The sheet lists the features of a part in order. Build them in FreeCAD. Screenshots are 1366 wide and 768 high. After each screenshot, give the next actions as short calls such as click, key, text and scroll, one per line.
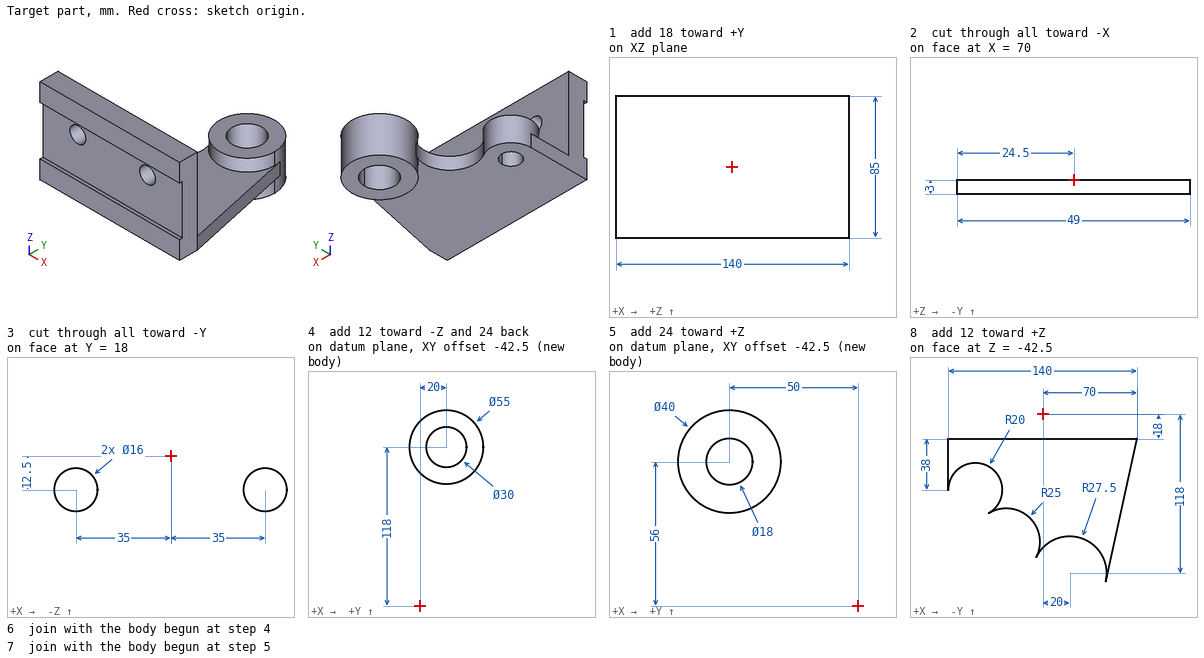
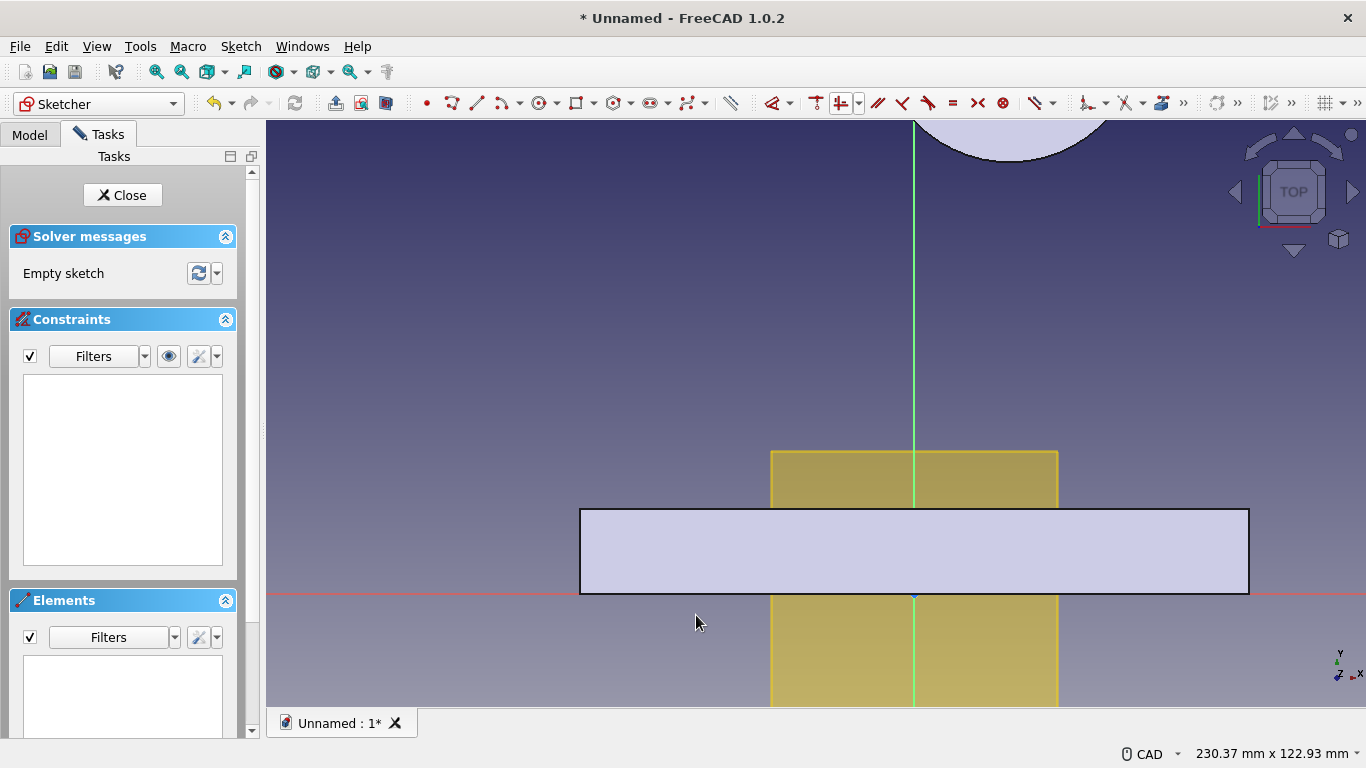
click(538, 104)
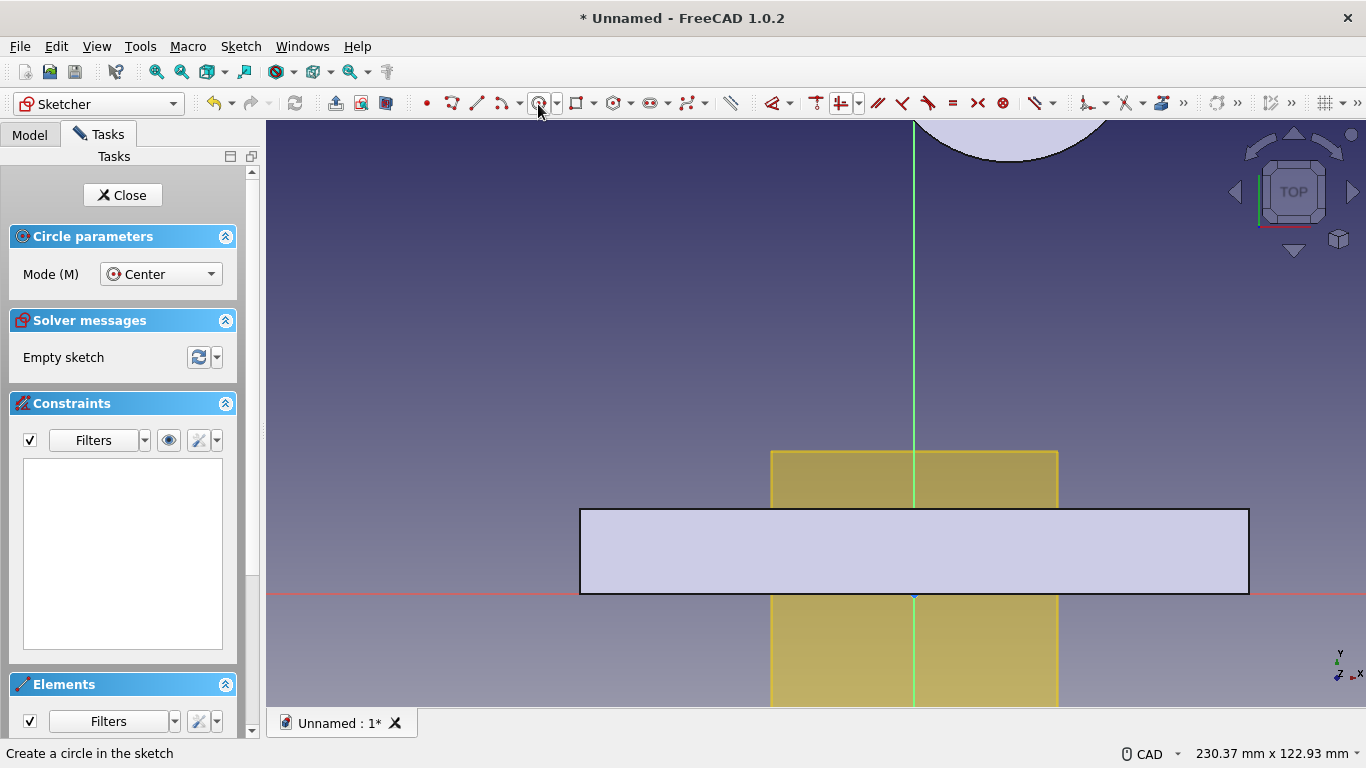
click(676, 327)
click(743, 260)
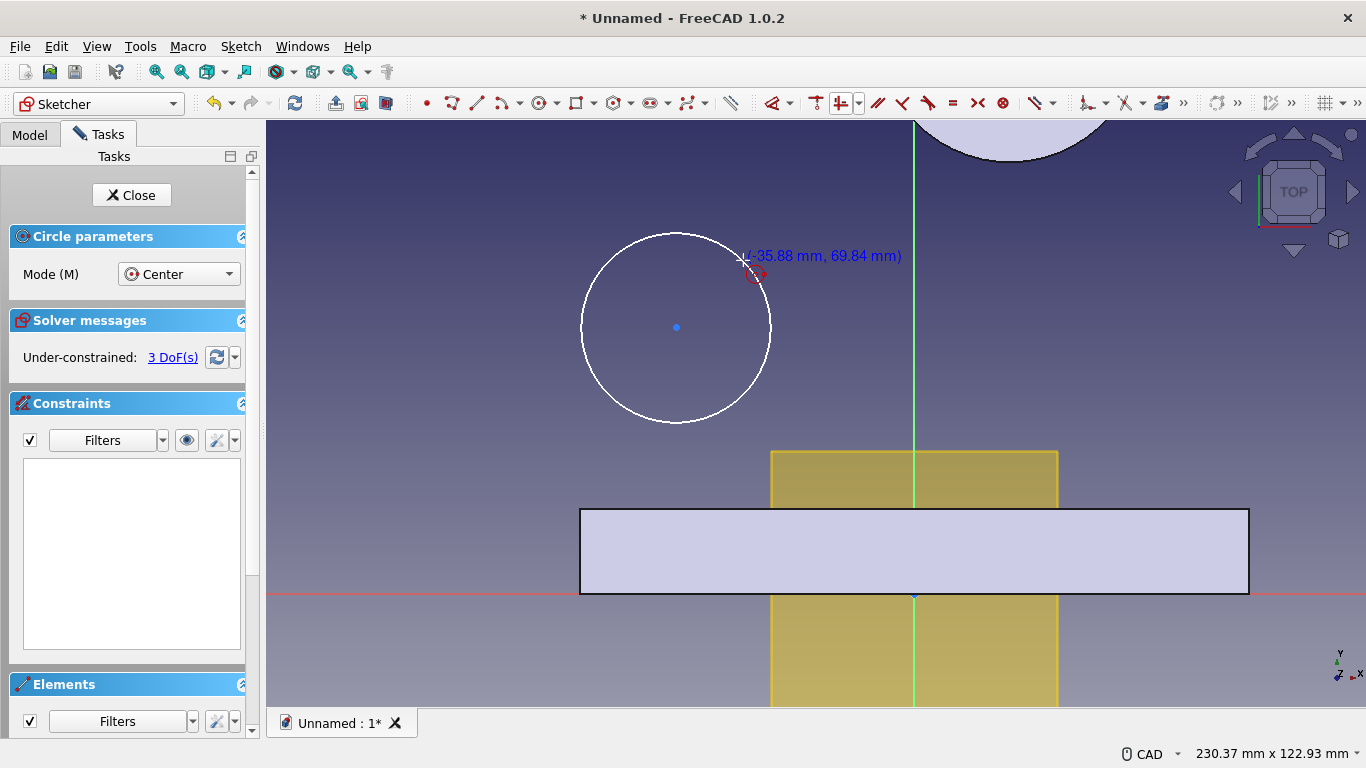
click(676, 328)
click(706, 297)
key(Escape)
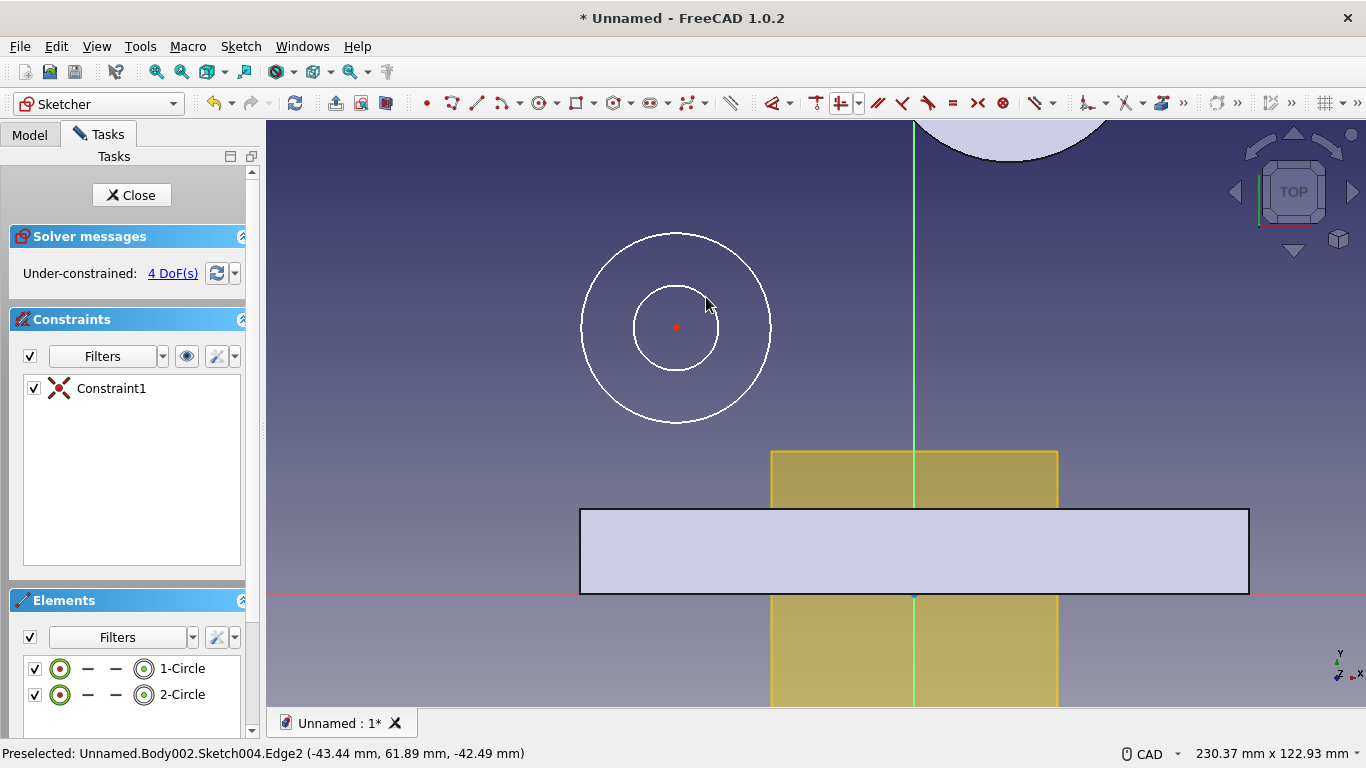
click(772, 104)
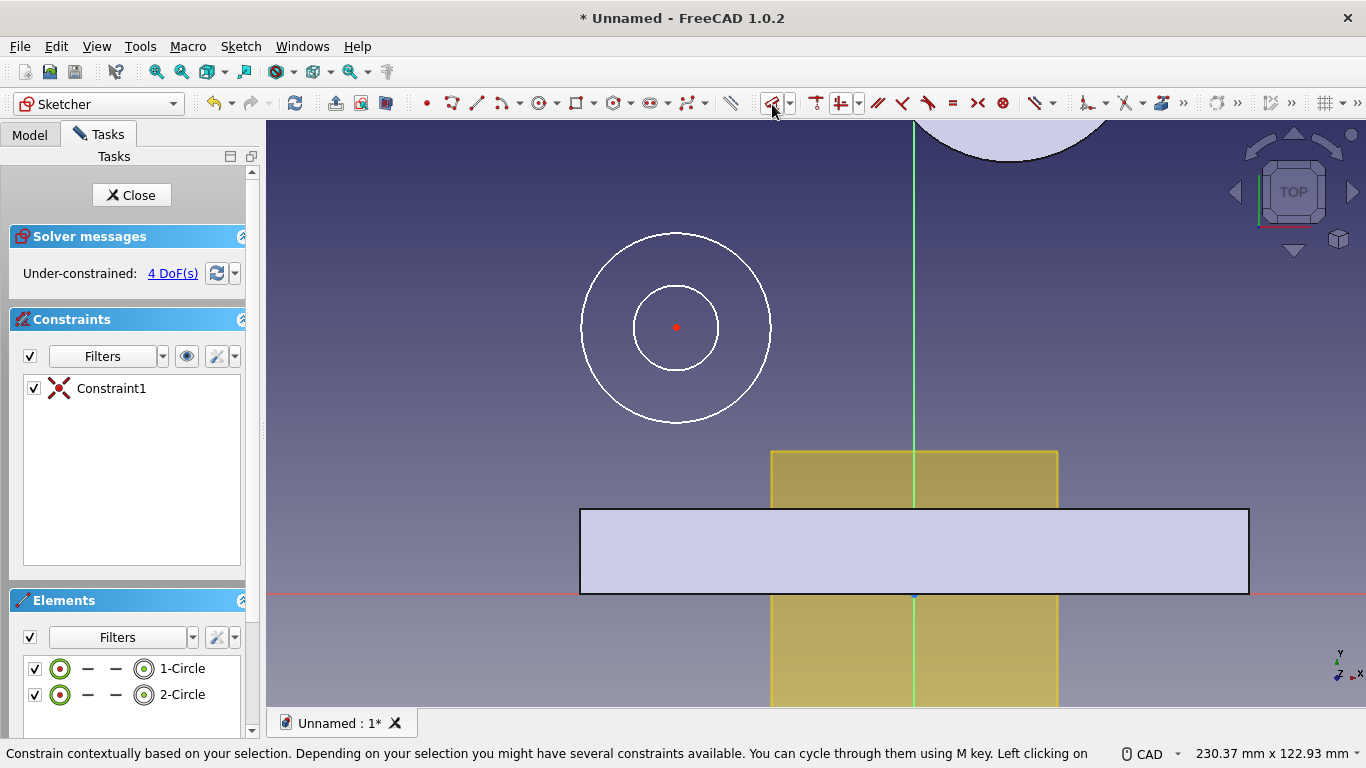
click(743, 261)
click(766, 238)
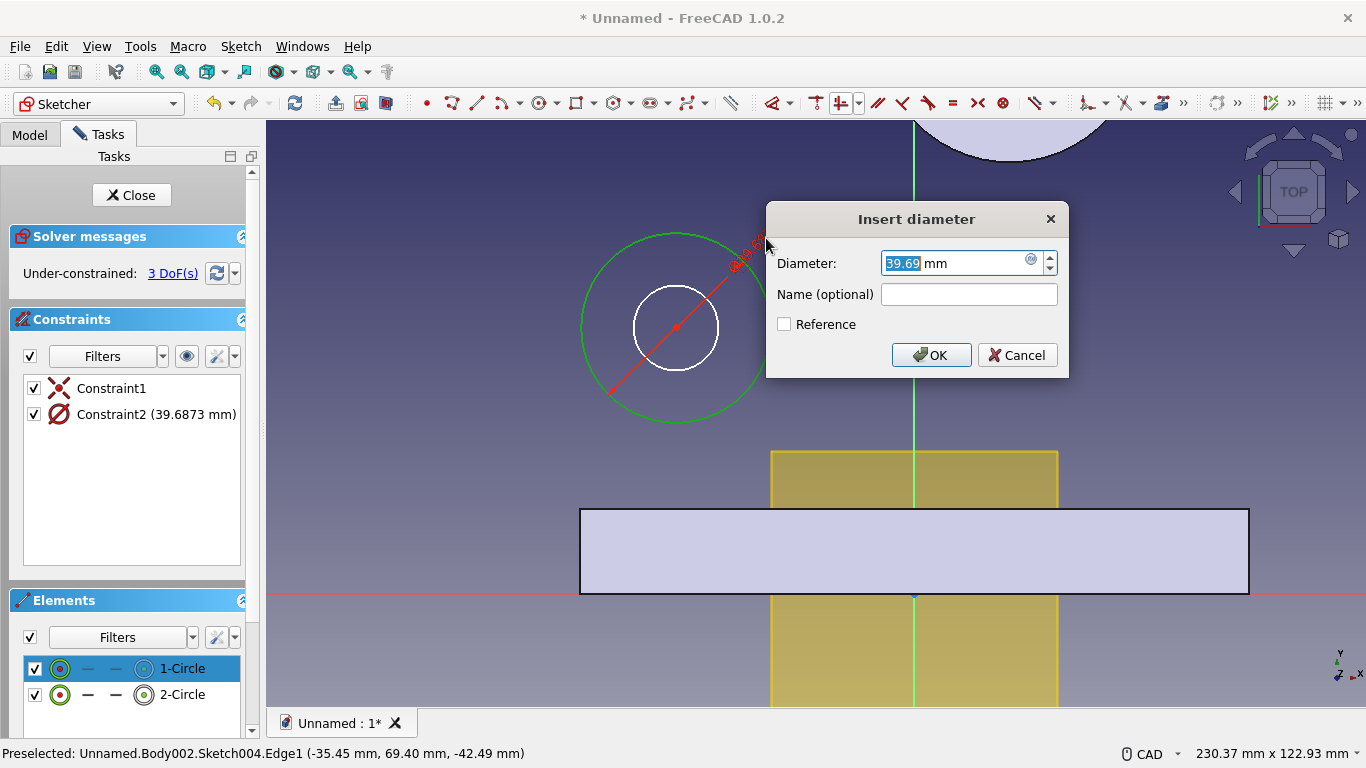
text(40)
key(Return)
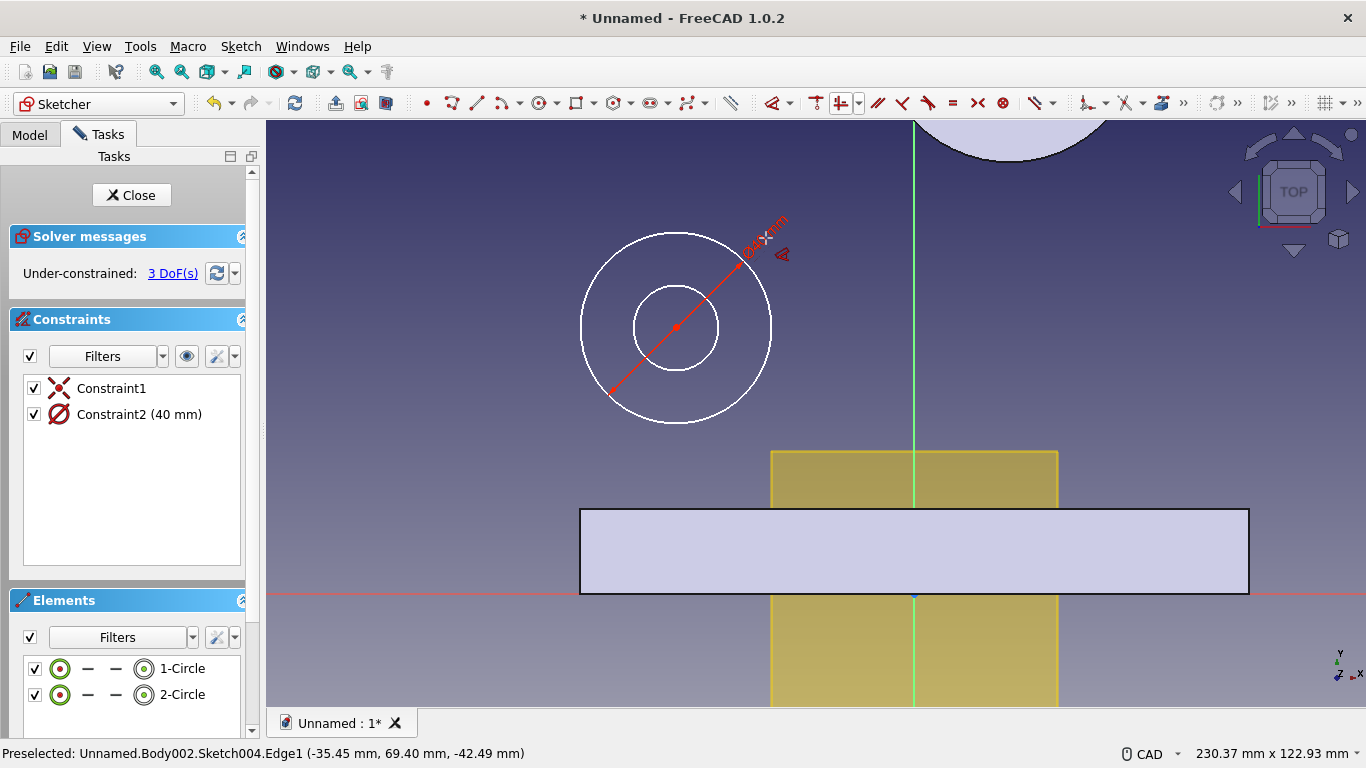
click(706, 298)
click(729, 275)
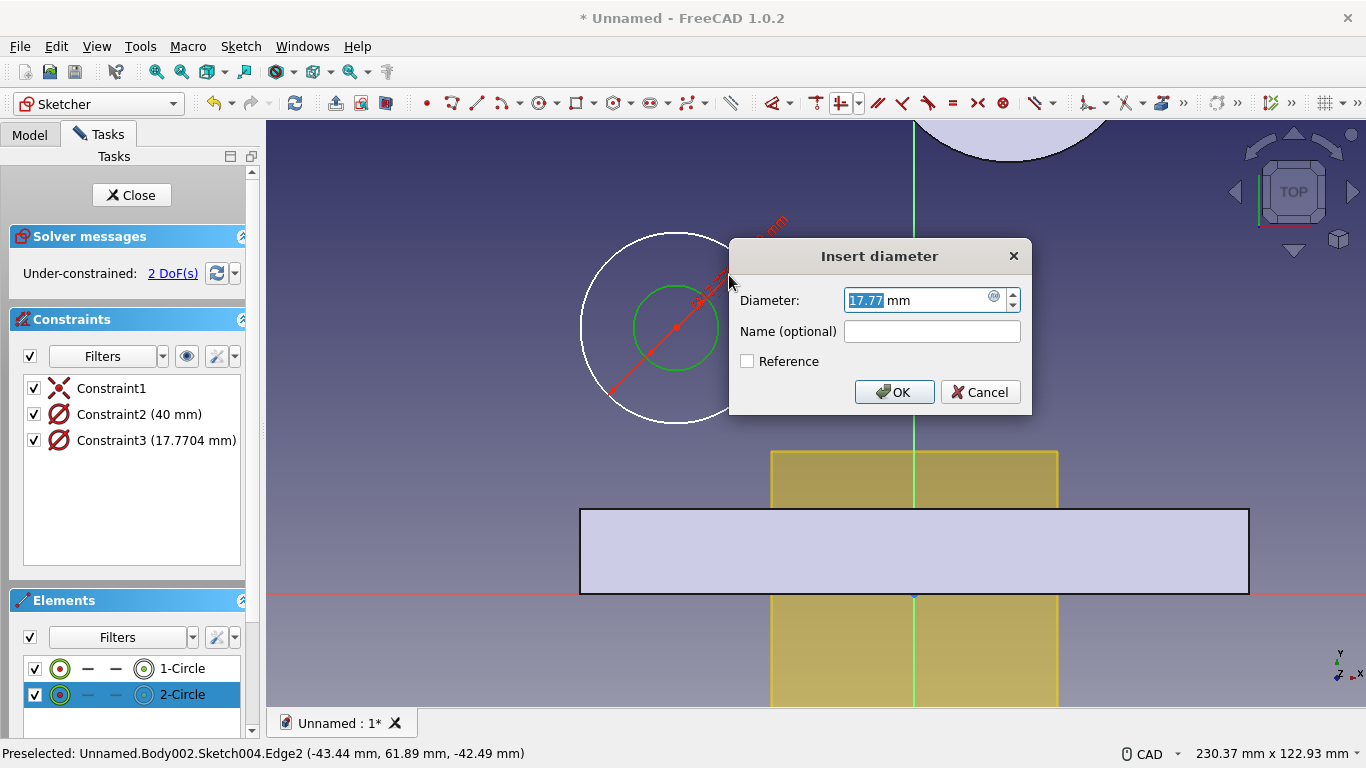
text(18)
key(Return)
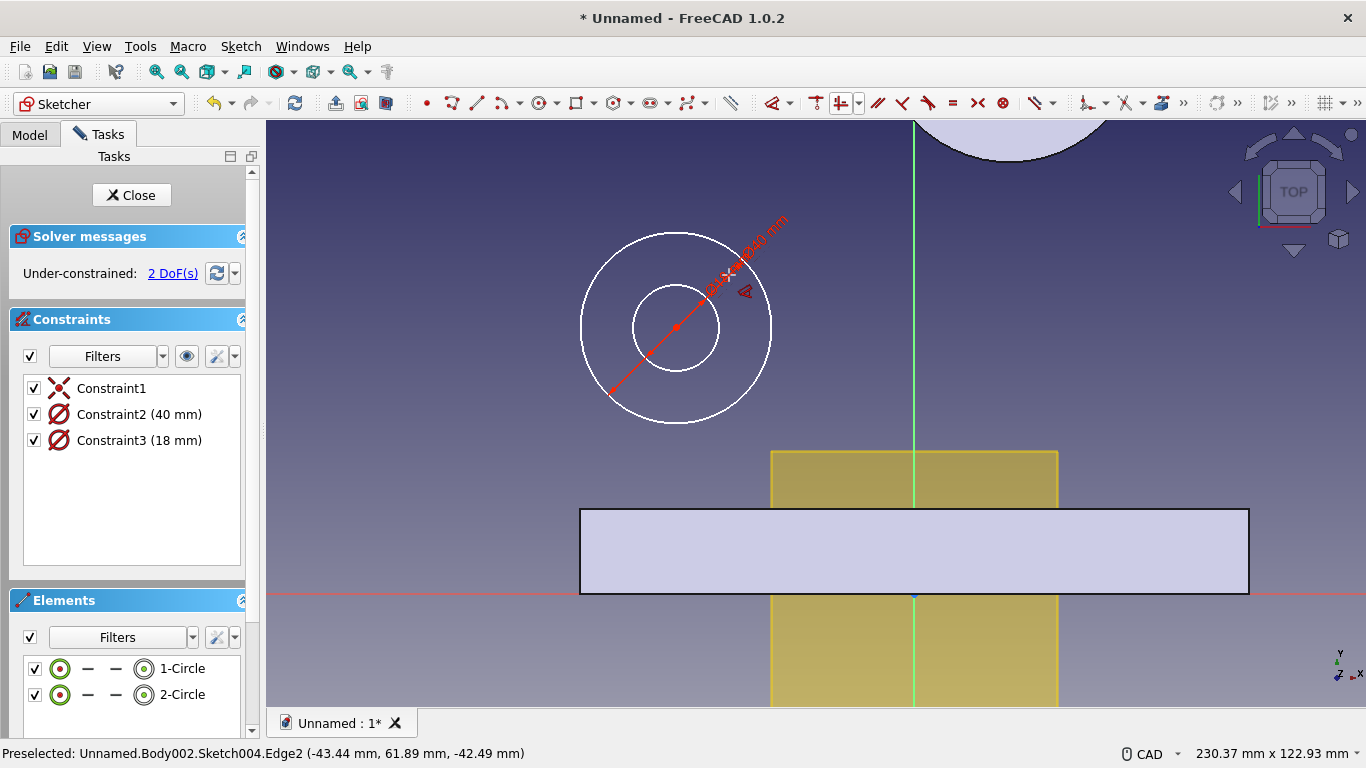
click(676, 328)
click(795, 628)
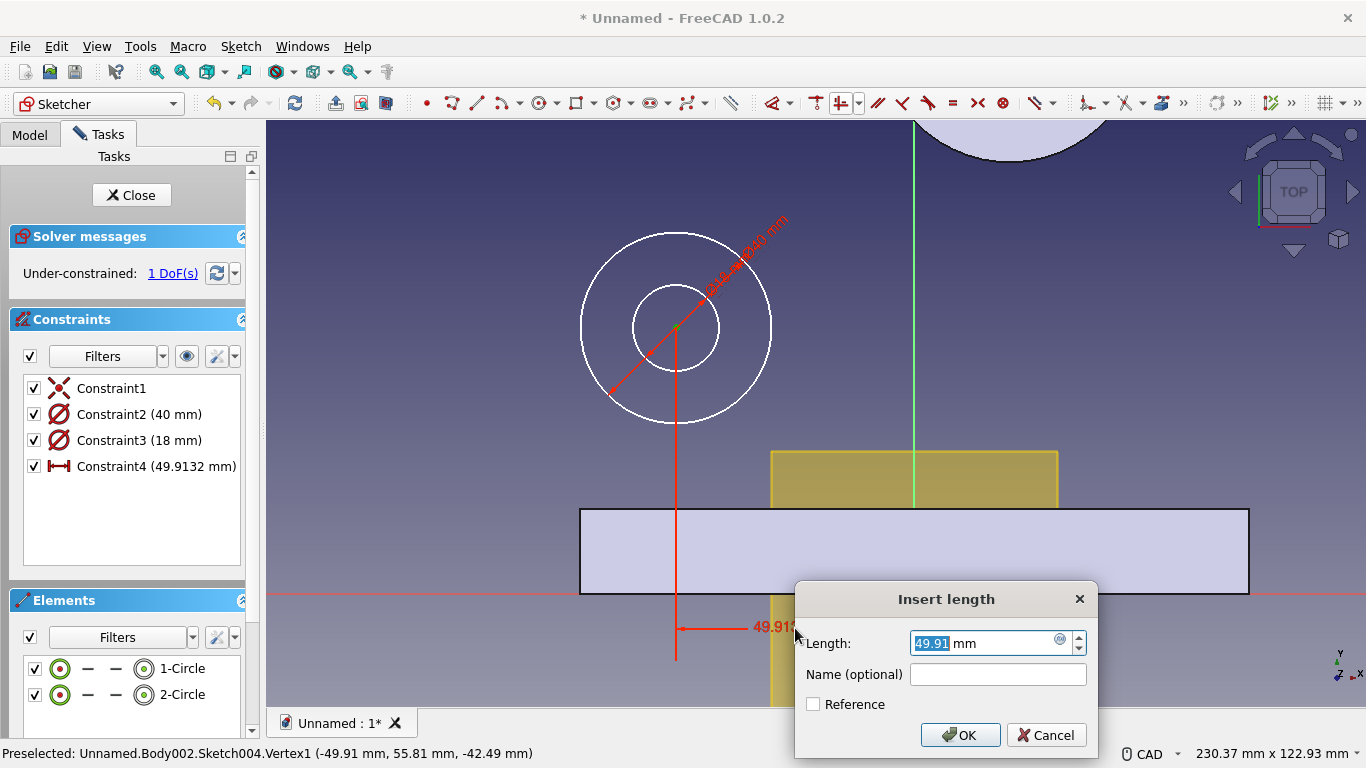
text(50)
key(Return)